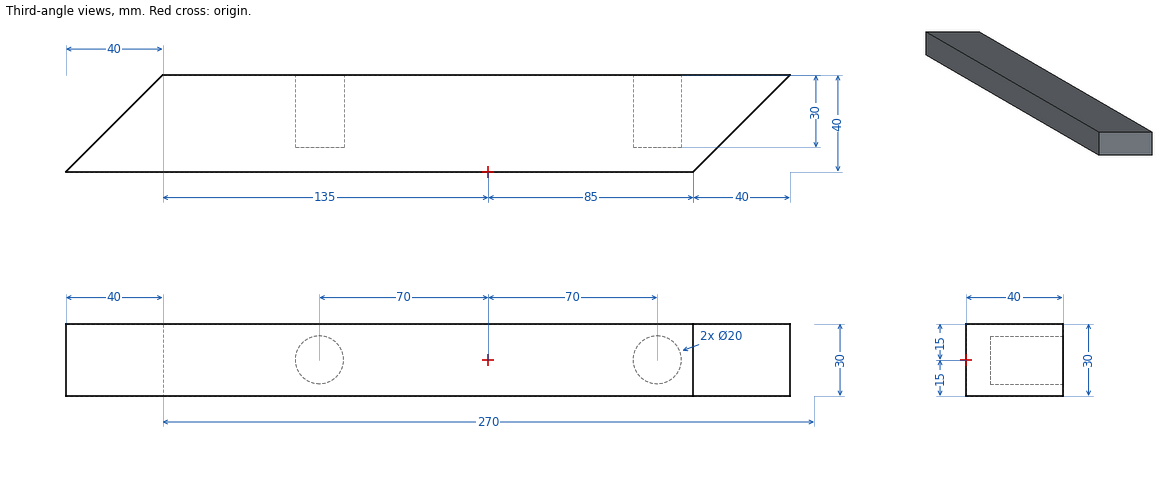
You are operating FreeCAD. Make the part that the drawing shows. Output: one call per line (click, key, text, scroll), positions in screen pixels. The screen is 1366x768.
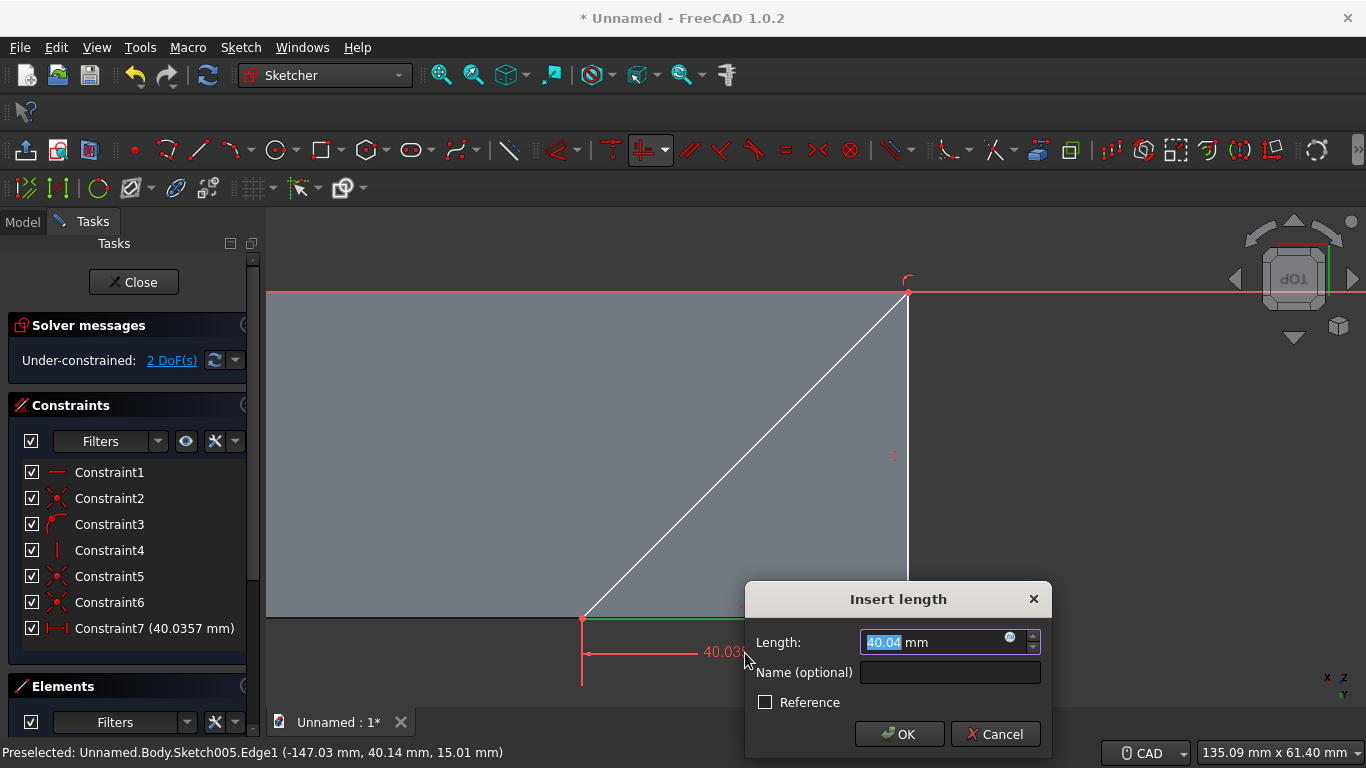
text(40)
key(Return)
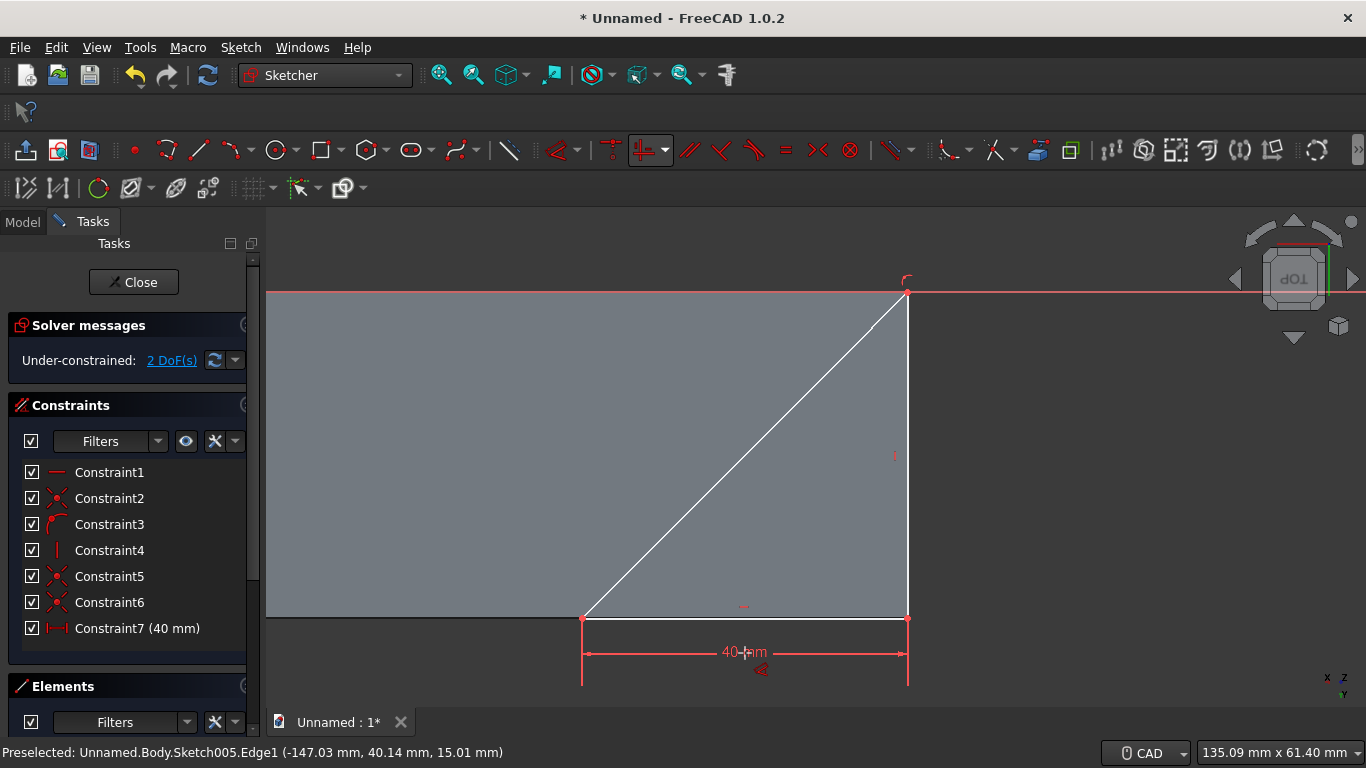
click(908, 521)
click(942, 456)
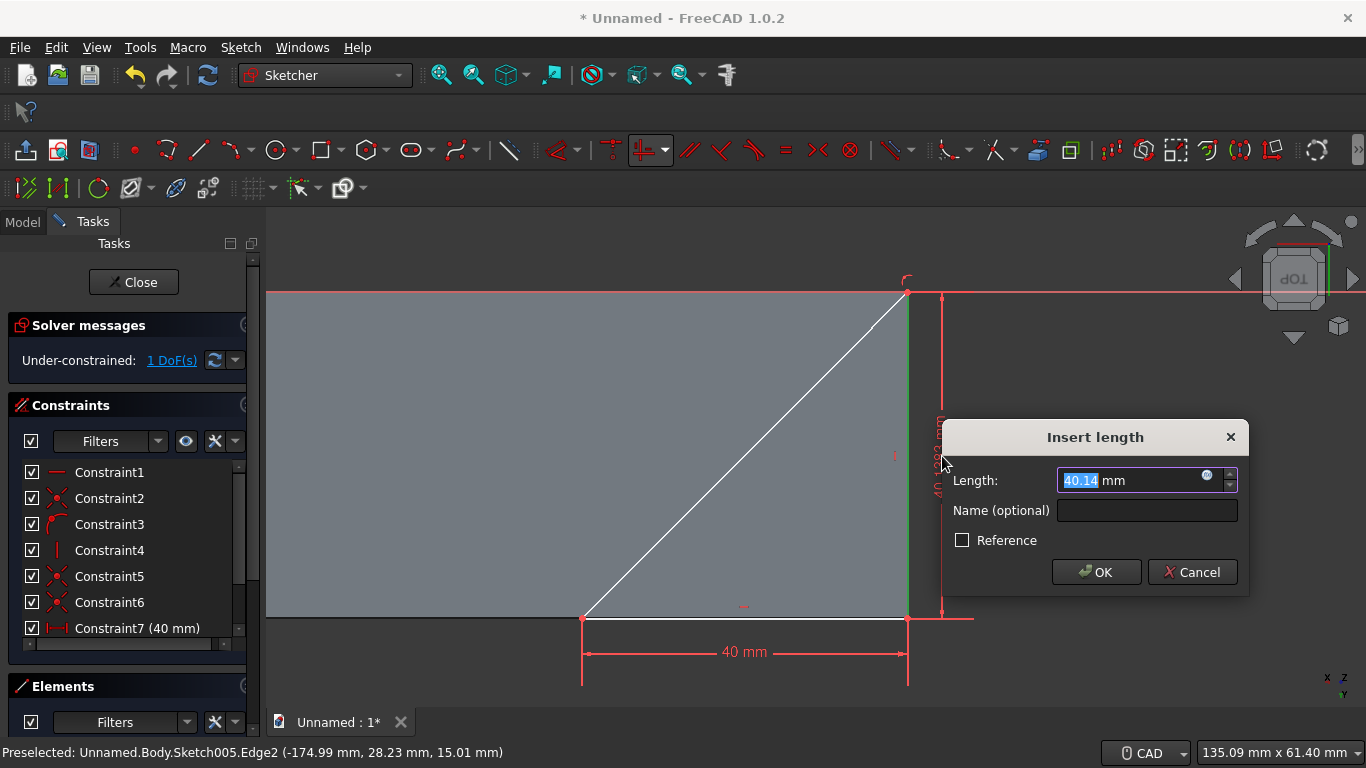
text(40)
key(Return)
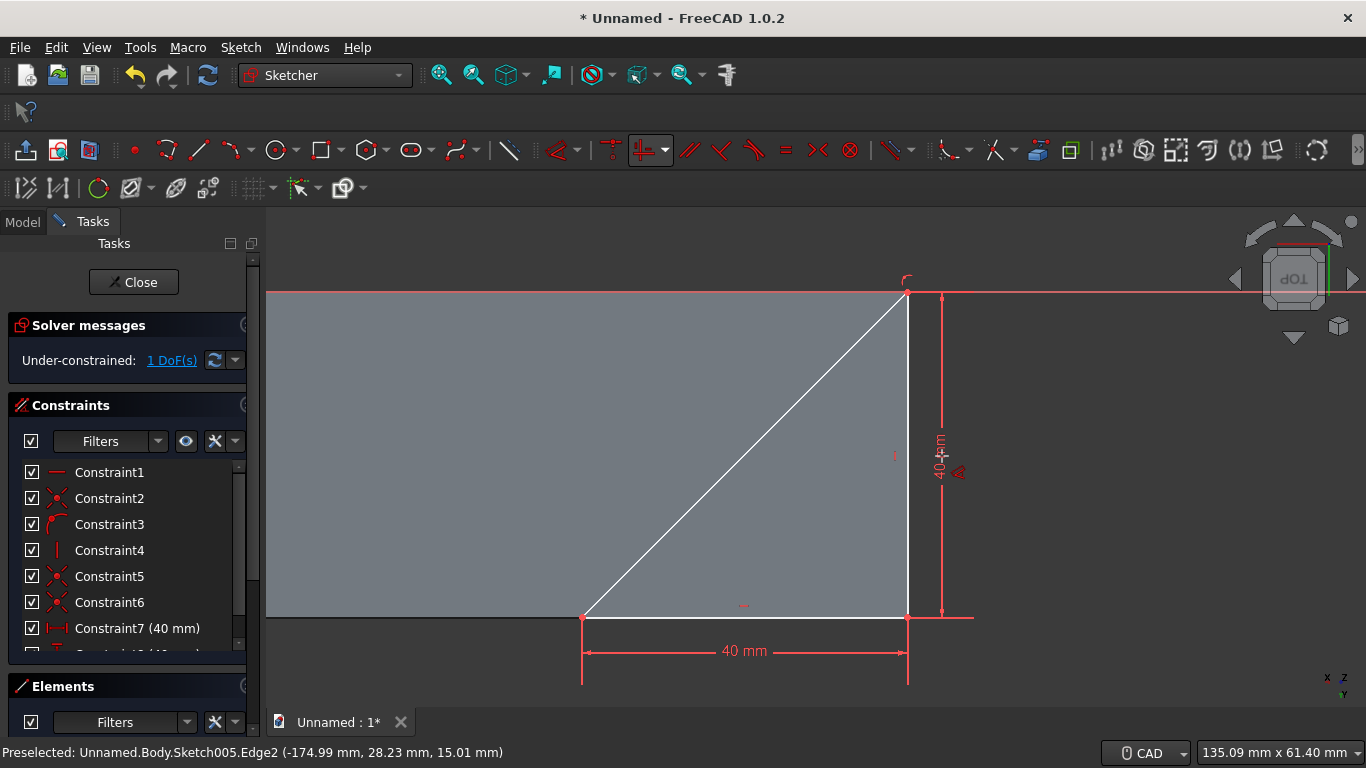
click(582, 618)
click(438, 652)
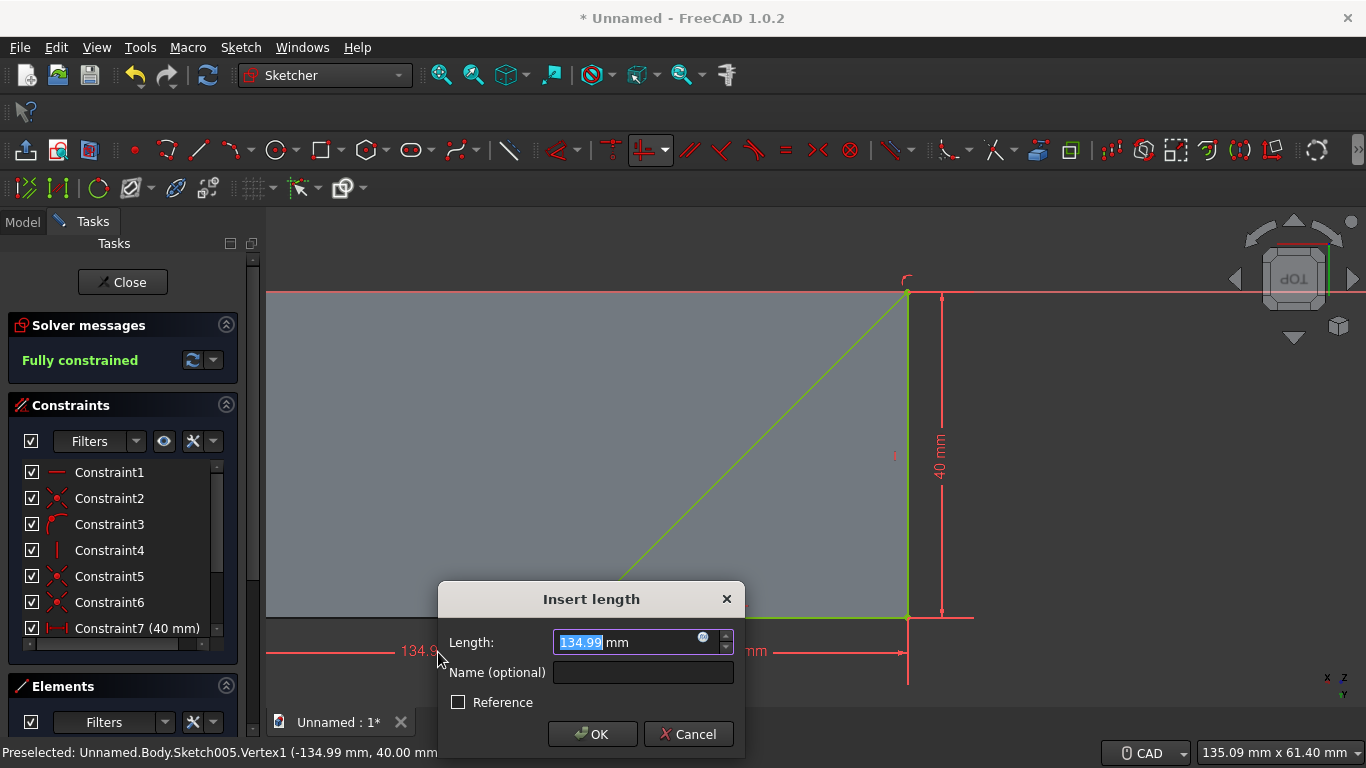
text(135)
key(Return)
key(Escape)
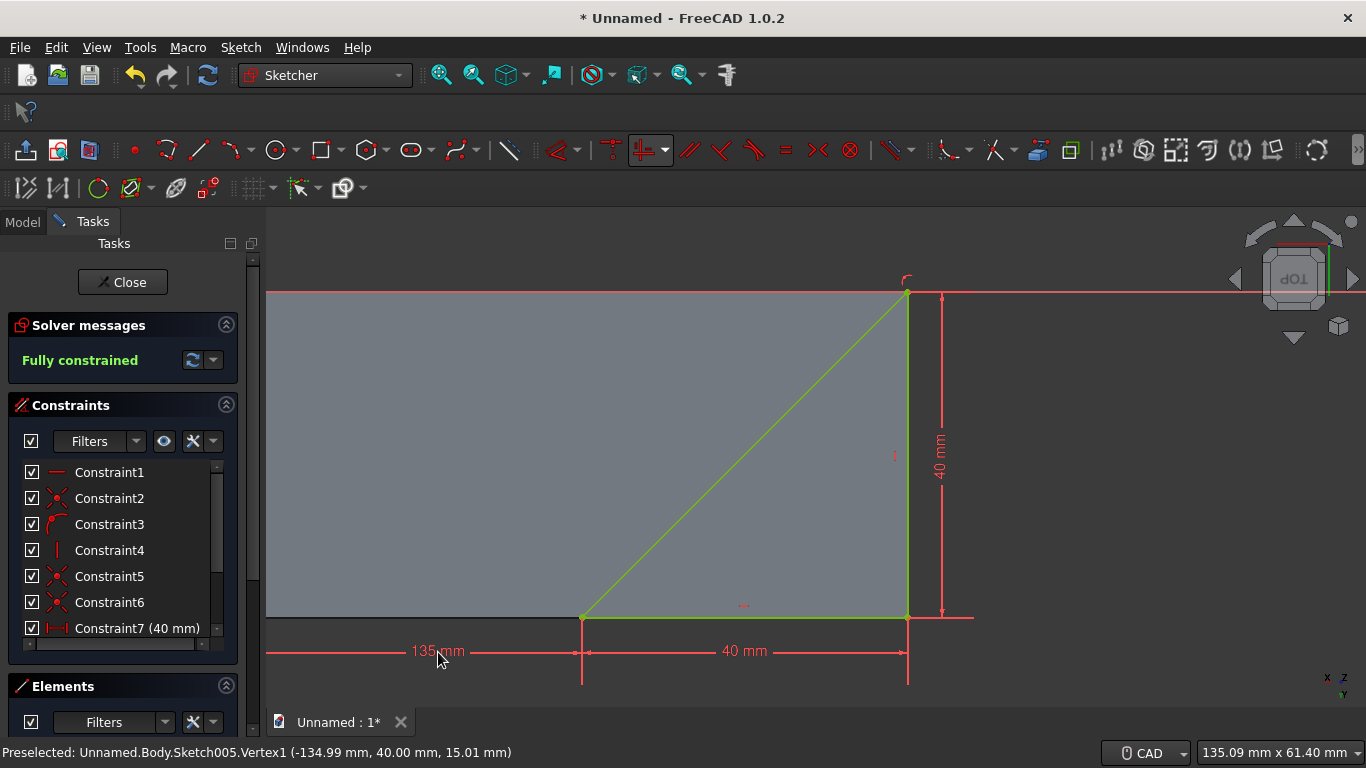
click(123, 282)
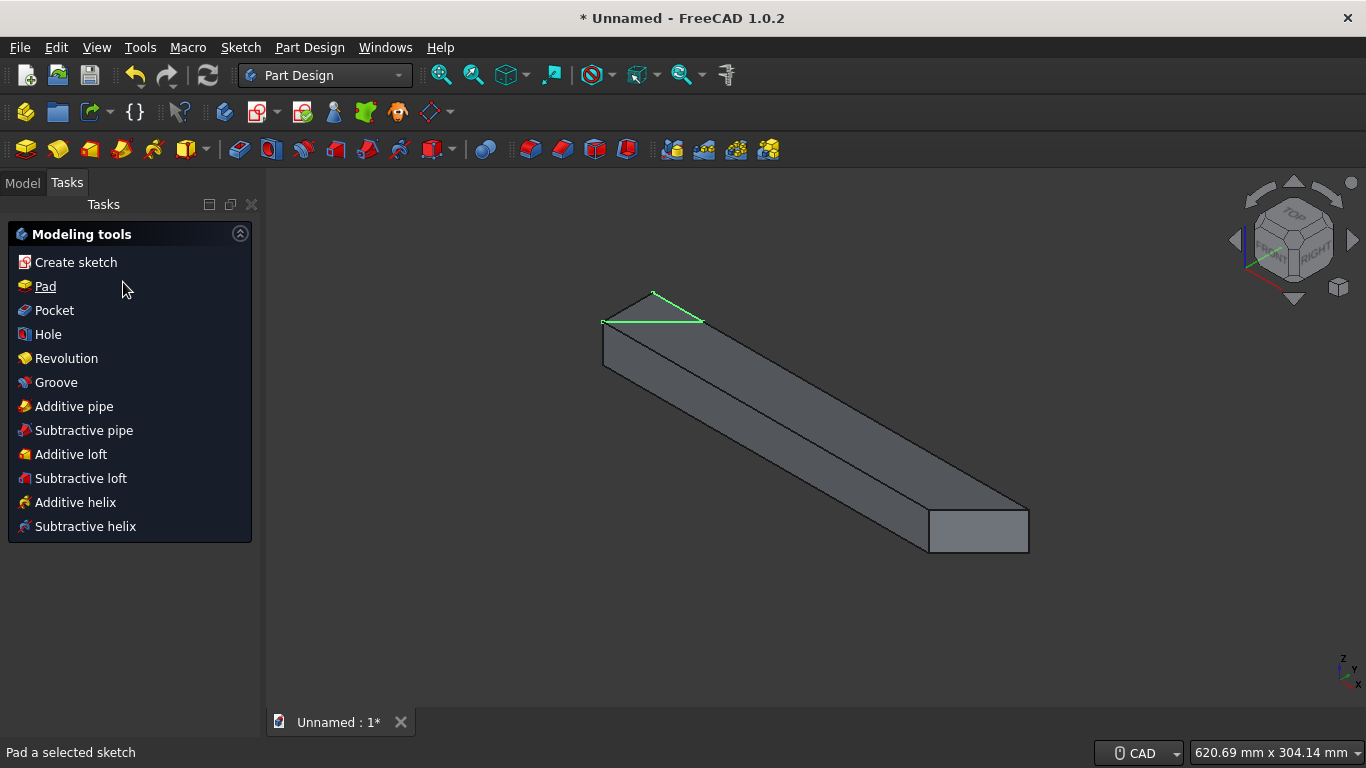
click(240, 150)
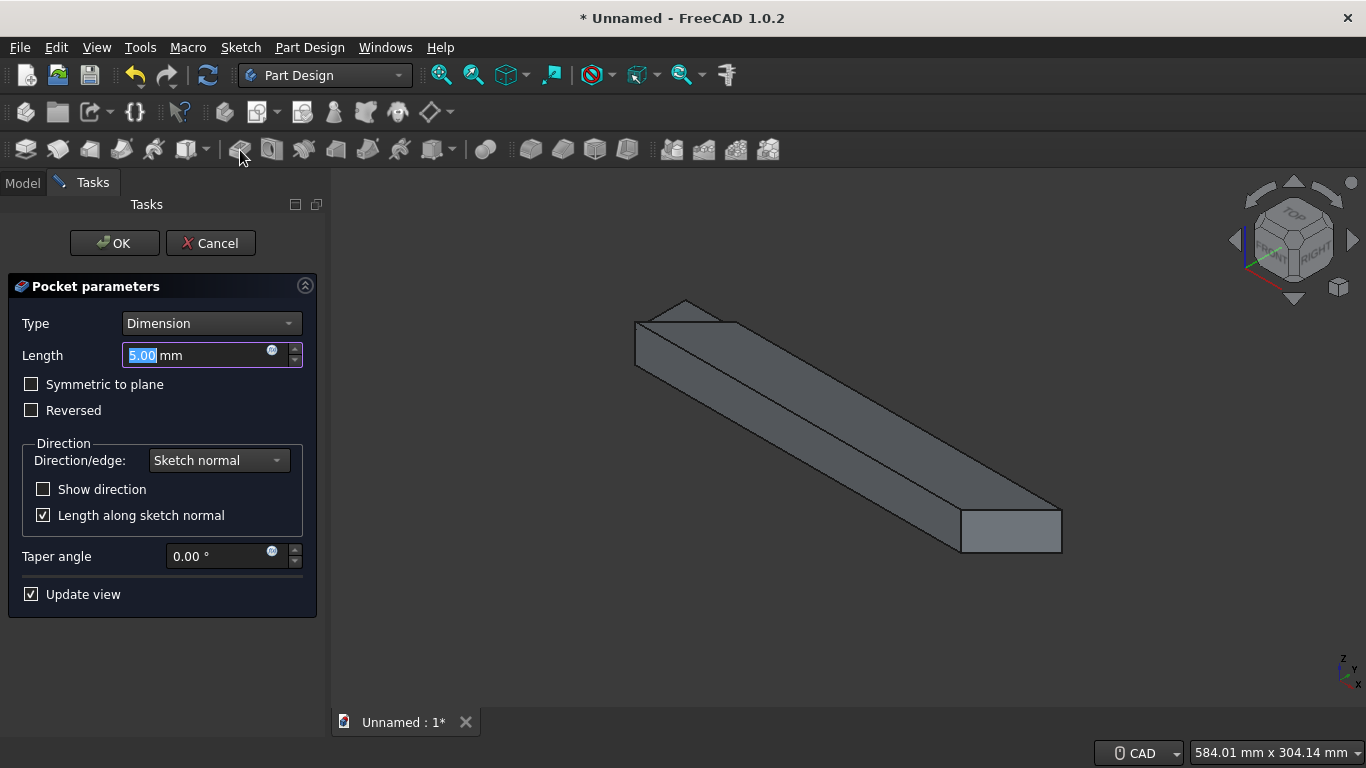
click(212, 324)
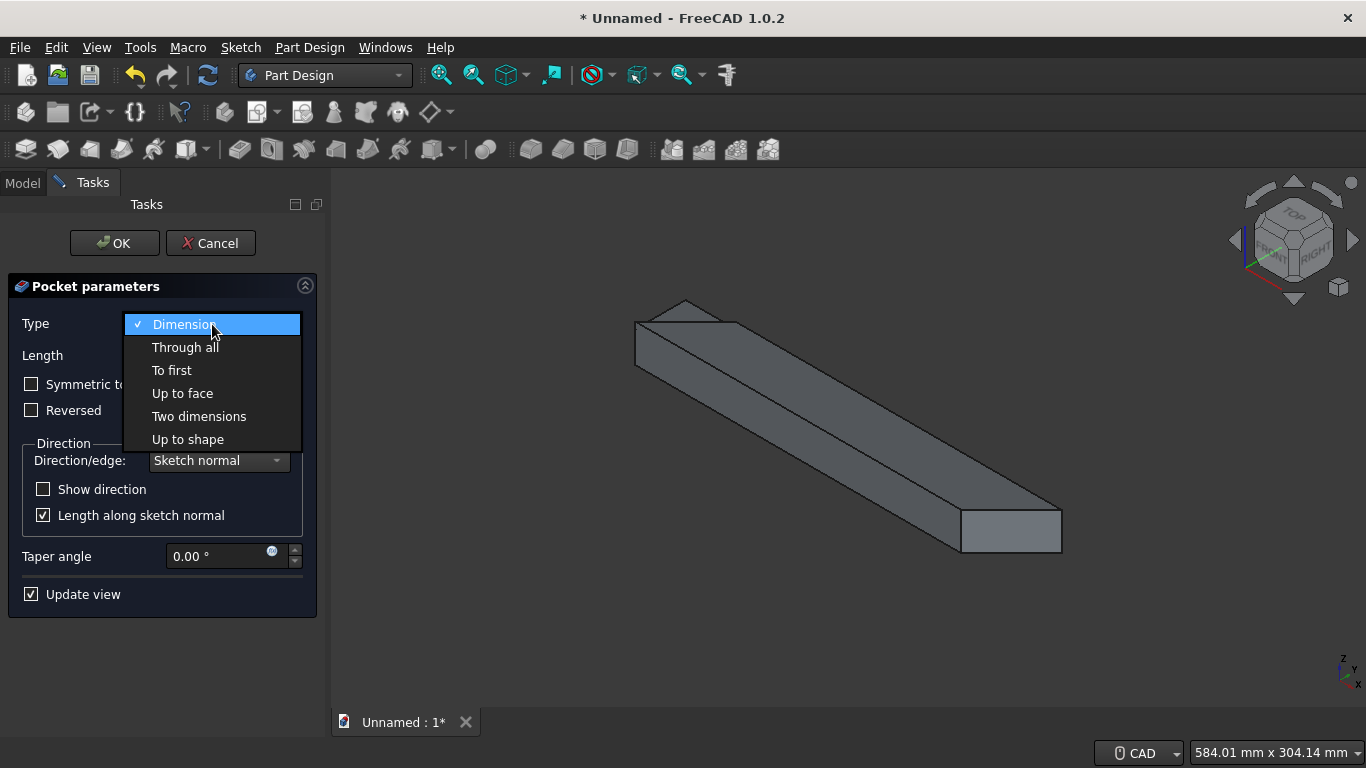
click(212, 348)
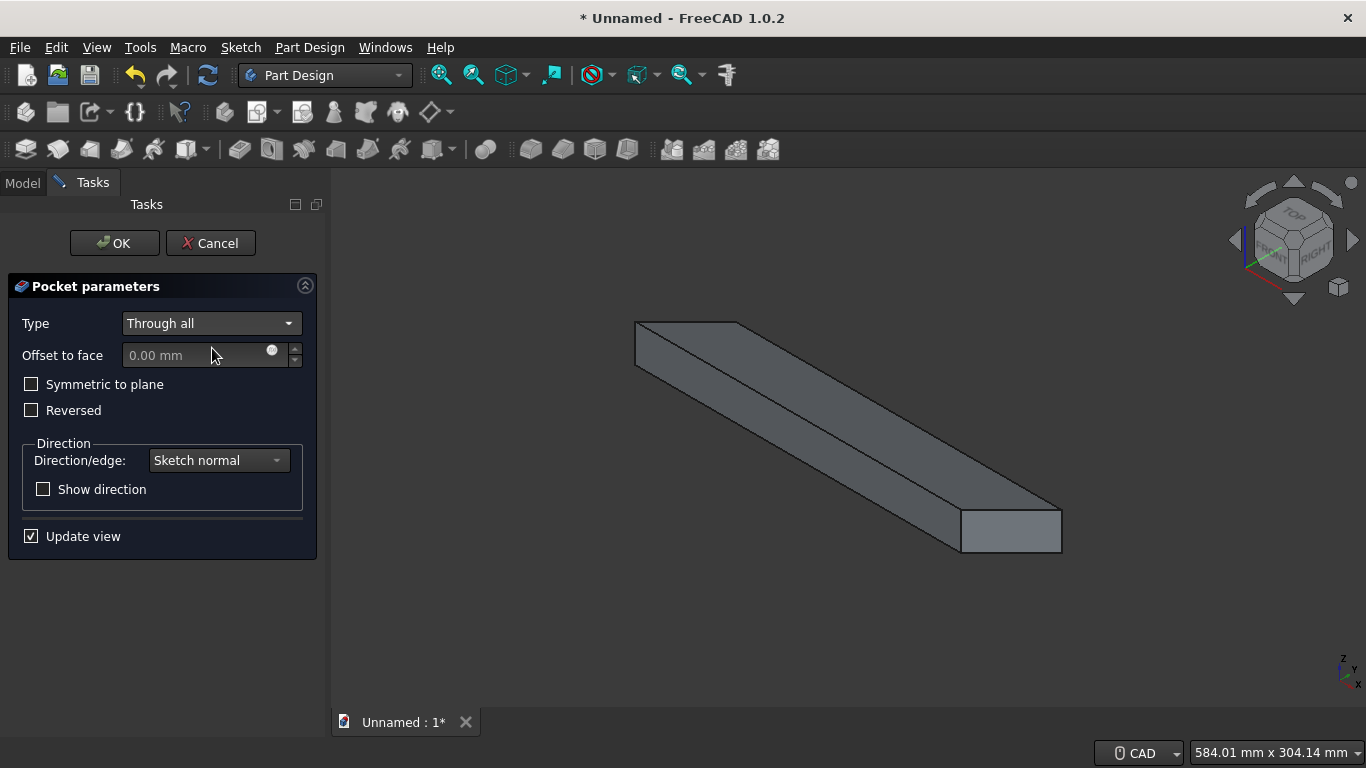
click(115, 243)